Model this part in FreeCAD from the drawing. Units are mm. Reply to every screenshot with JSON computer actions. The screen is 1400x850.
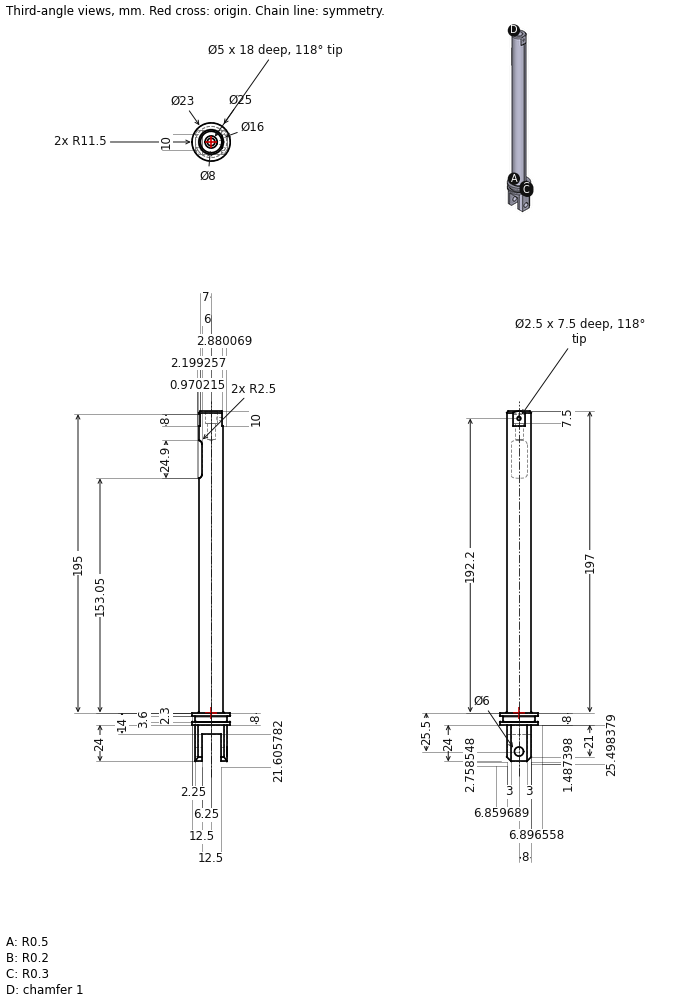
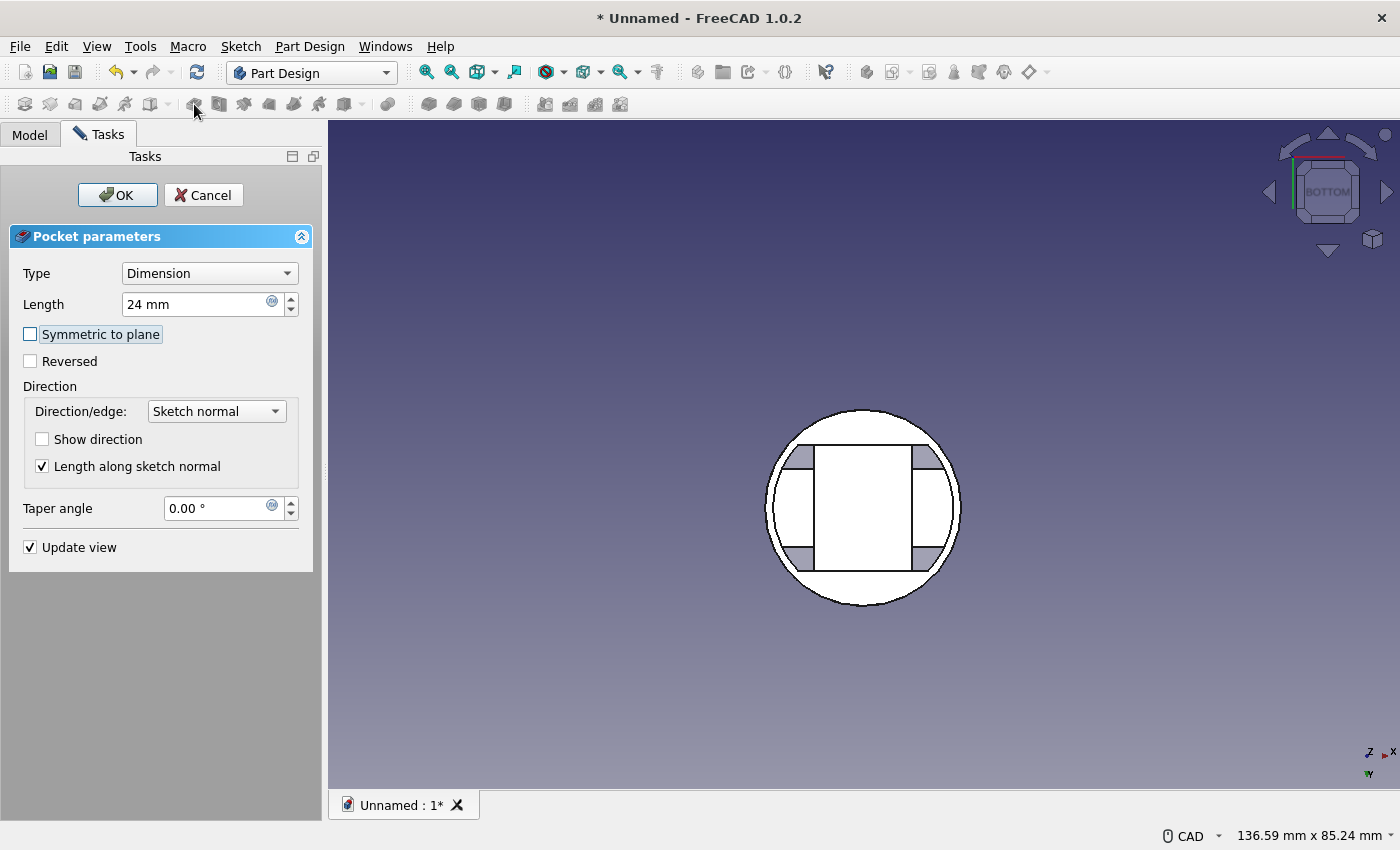
{"action": "left_click", "coordinate": [31, 361]}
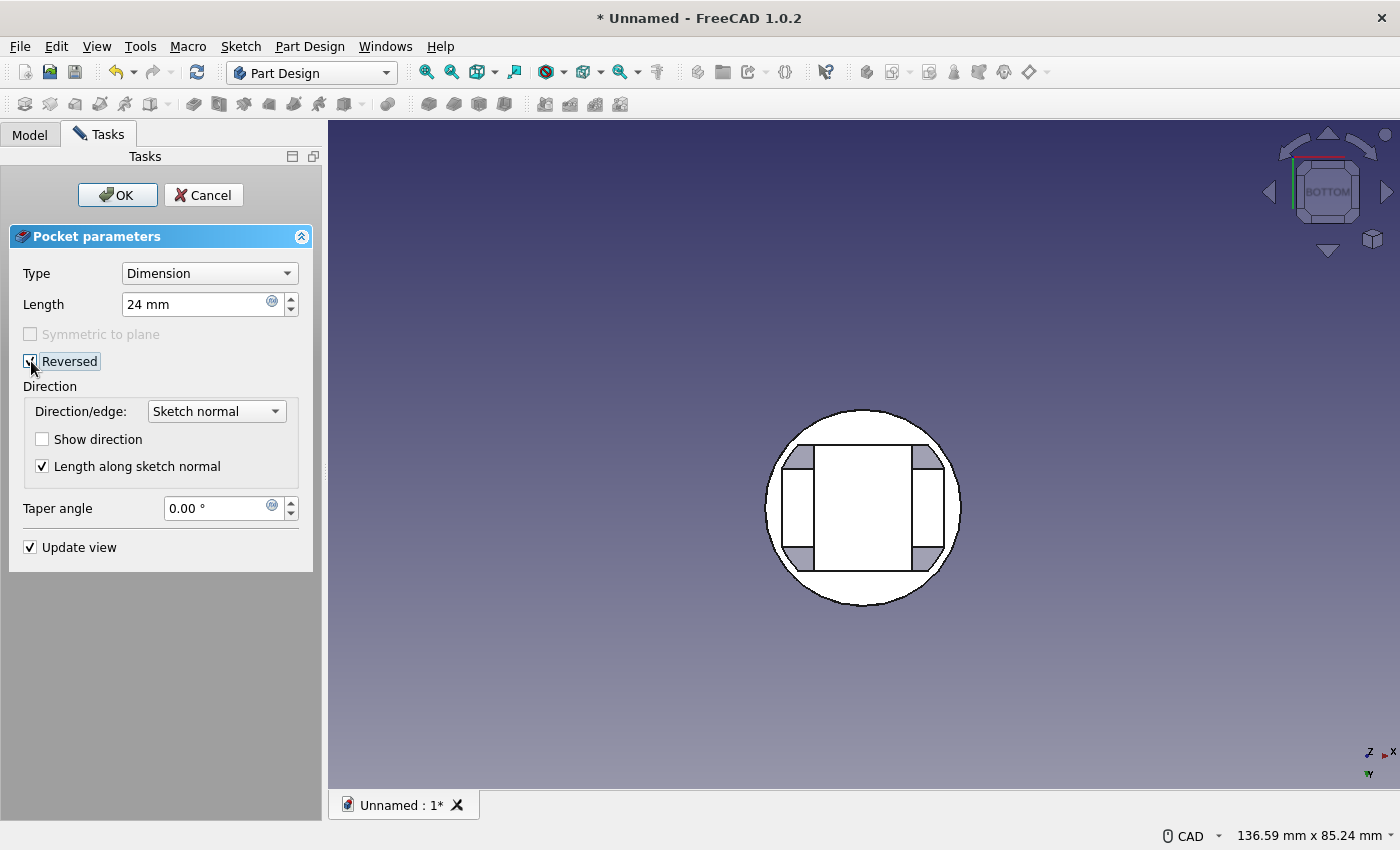
{"action": "left_click", "coordinate": [118, 195]}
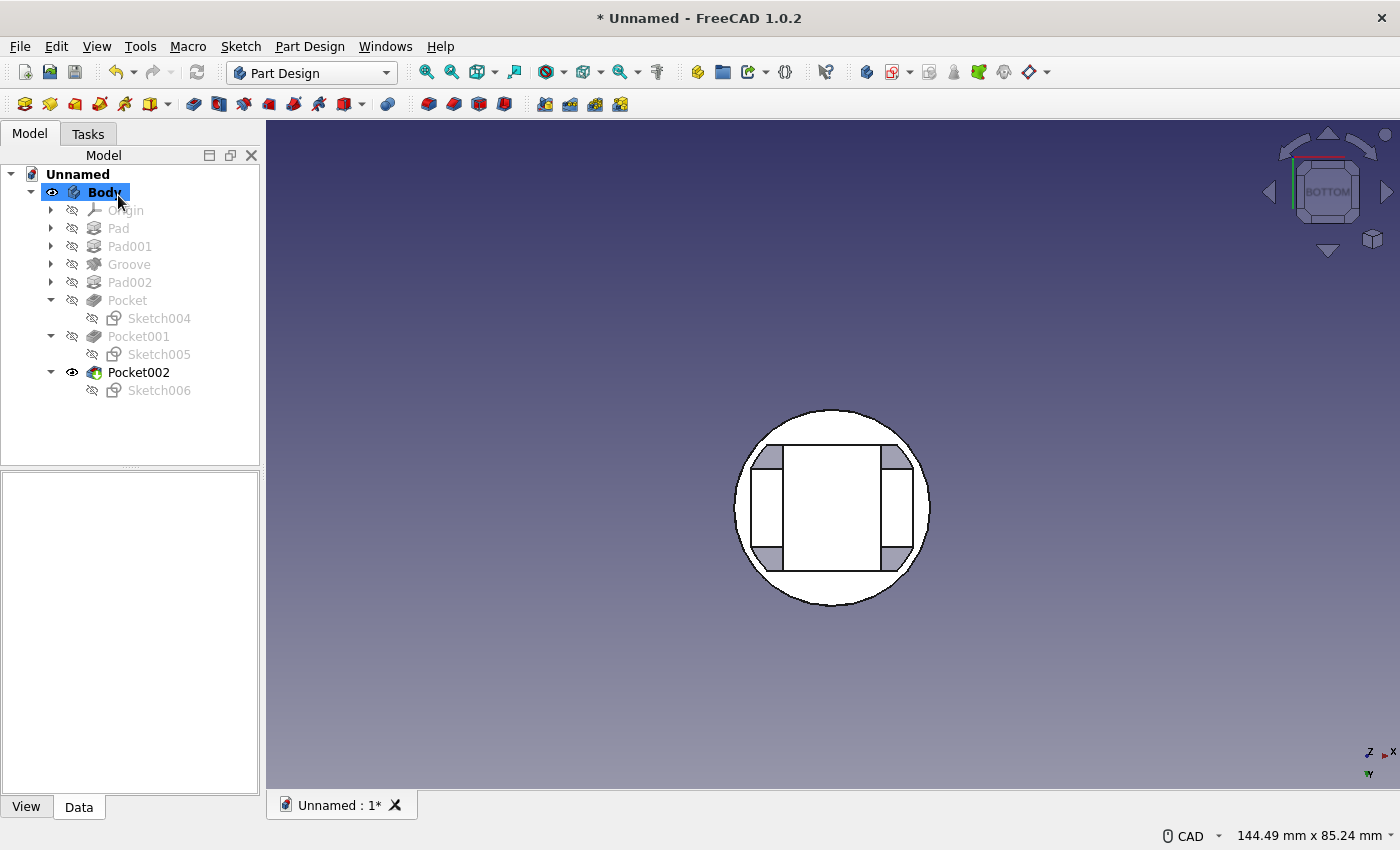
{"action": "left_click", "coordinate": [427, 72]}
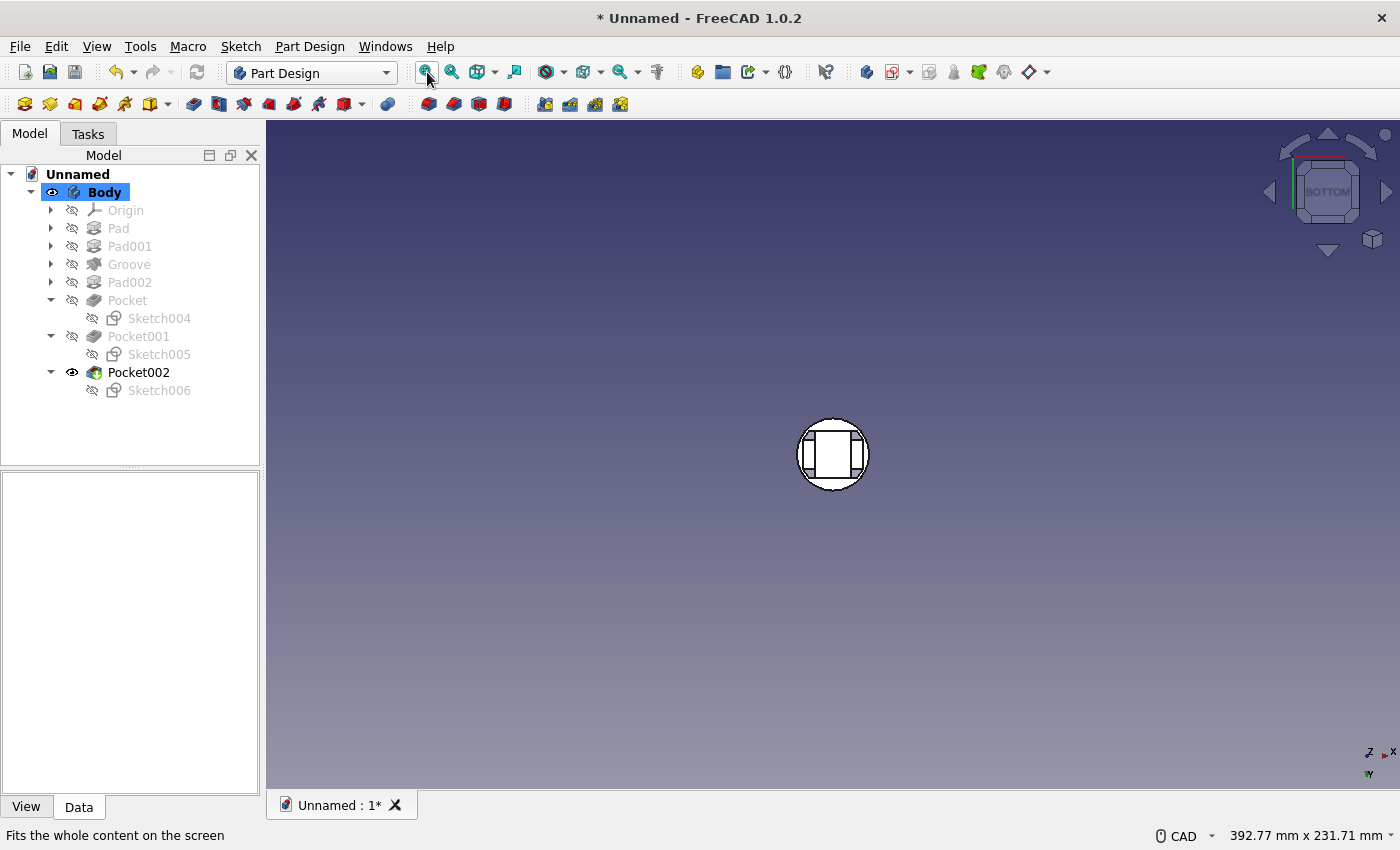
{"action": "key", "text": "0"}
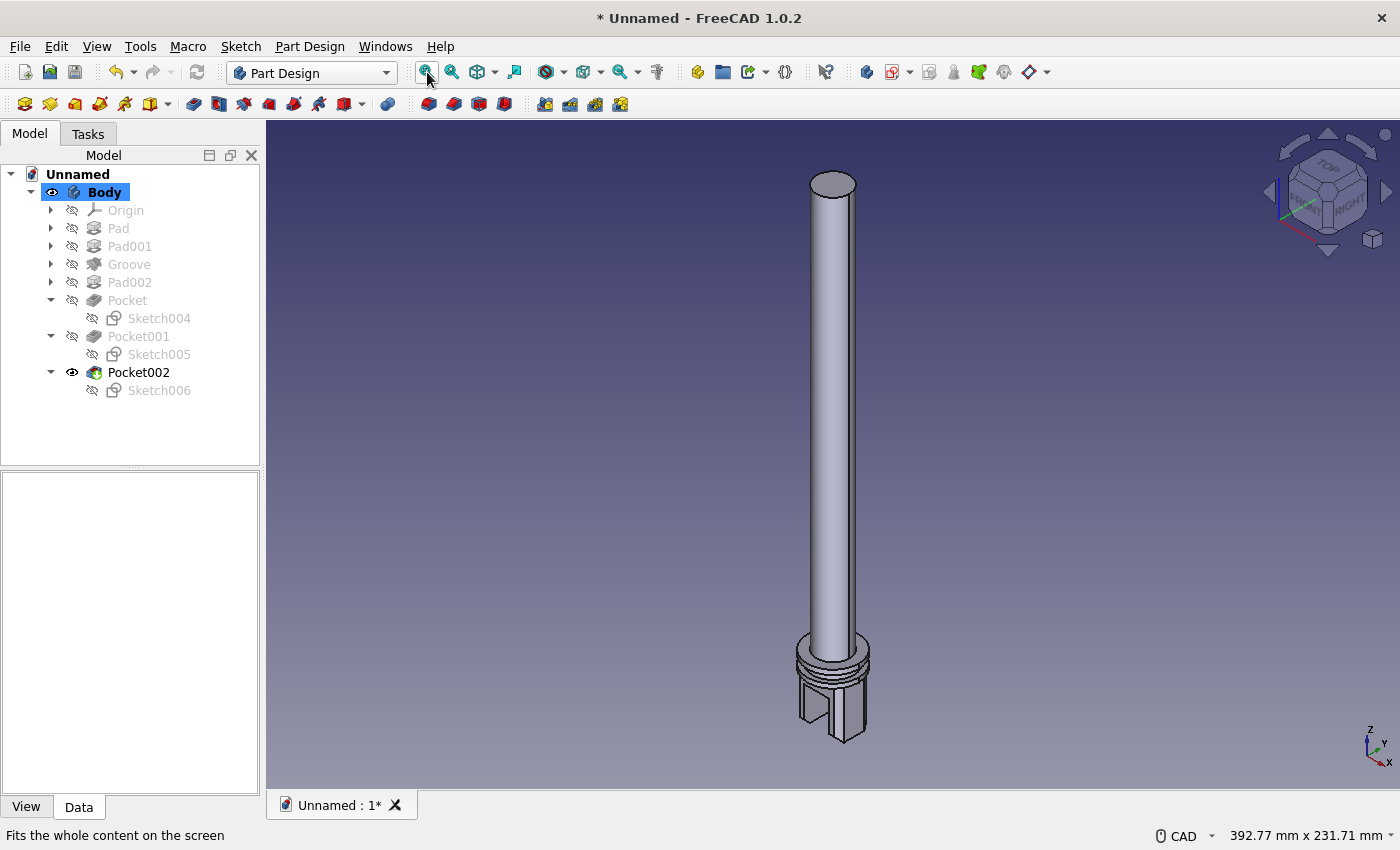
{"action": "left_click", "coordinate": [812, 654]}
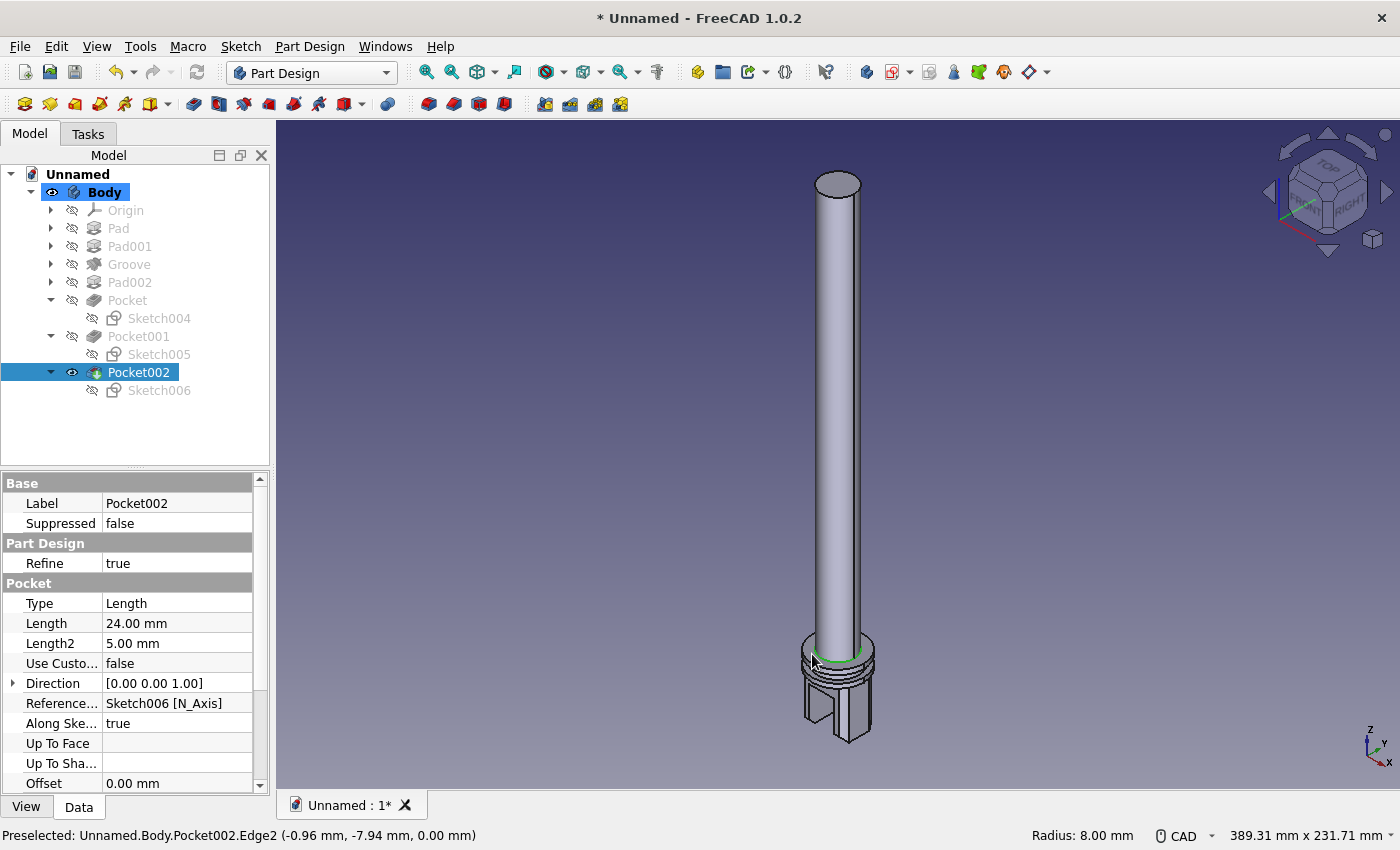
{"action": "left_click", "coordinate": [429, 104]}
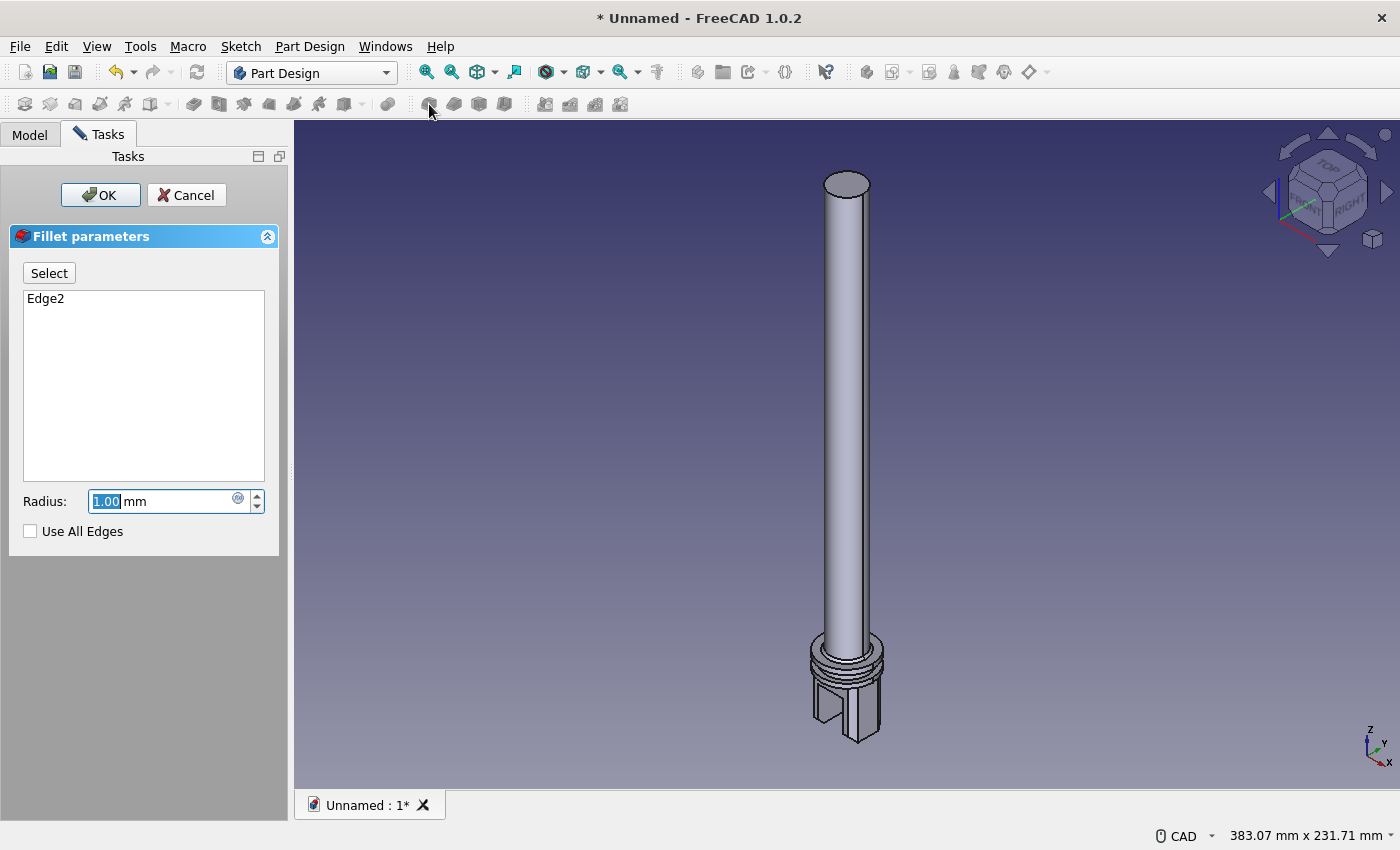
{"action": "type", "text": "0.5"}
{"action": "key", "text": "Tab"}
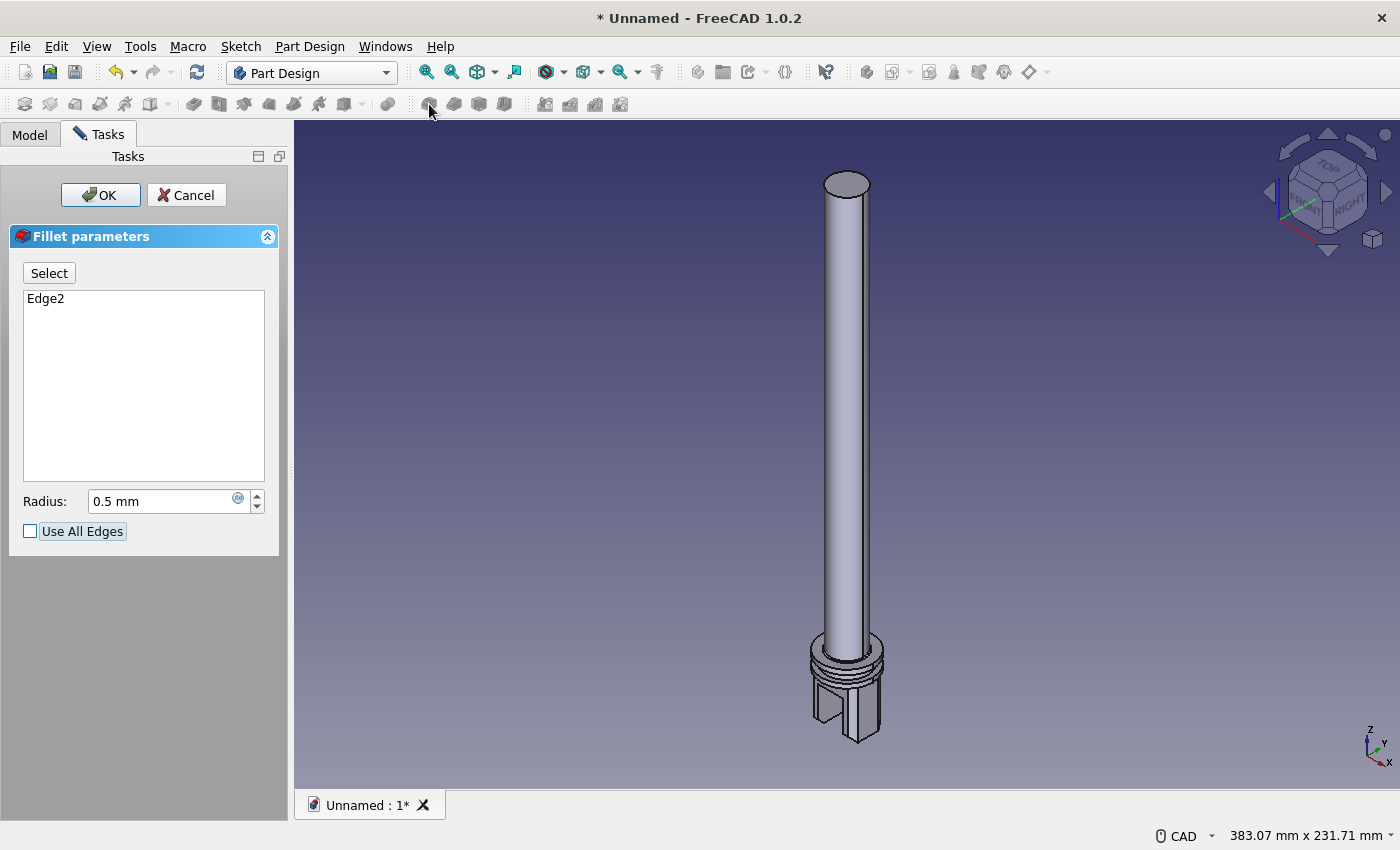
{"action": "left_click", "coordinate": [101, 195]}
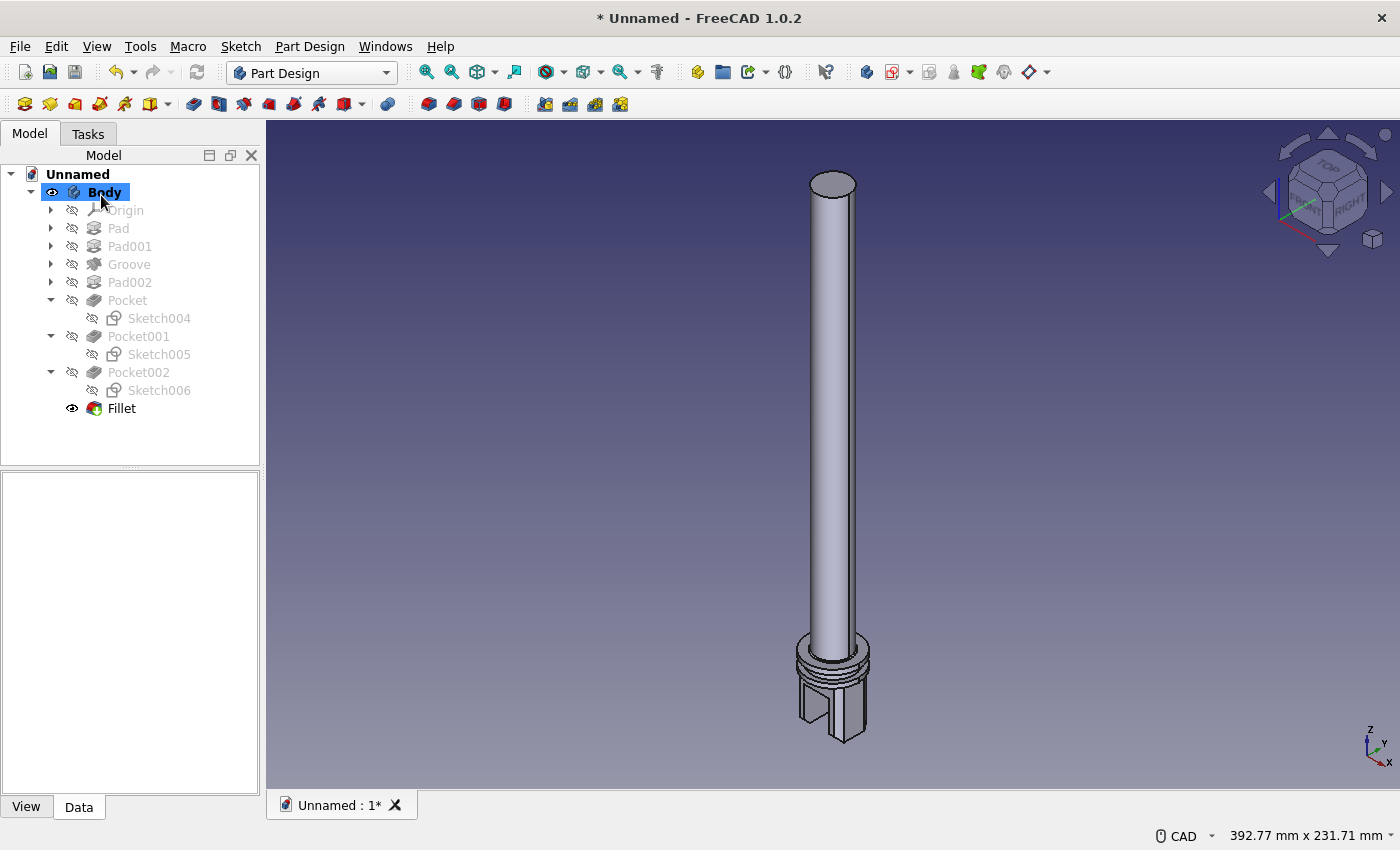
{"action": "key", "text": "2"}